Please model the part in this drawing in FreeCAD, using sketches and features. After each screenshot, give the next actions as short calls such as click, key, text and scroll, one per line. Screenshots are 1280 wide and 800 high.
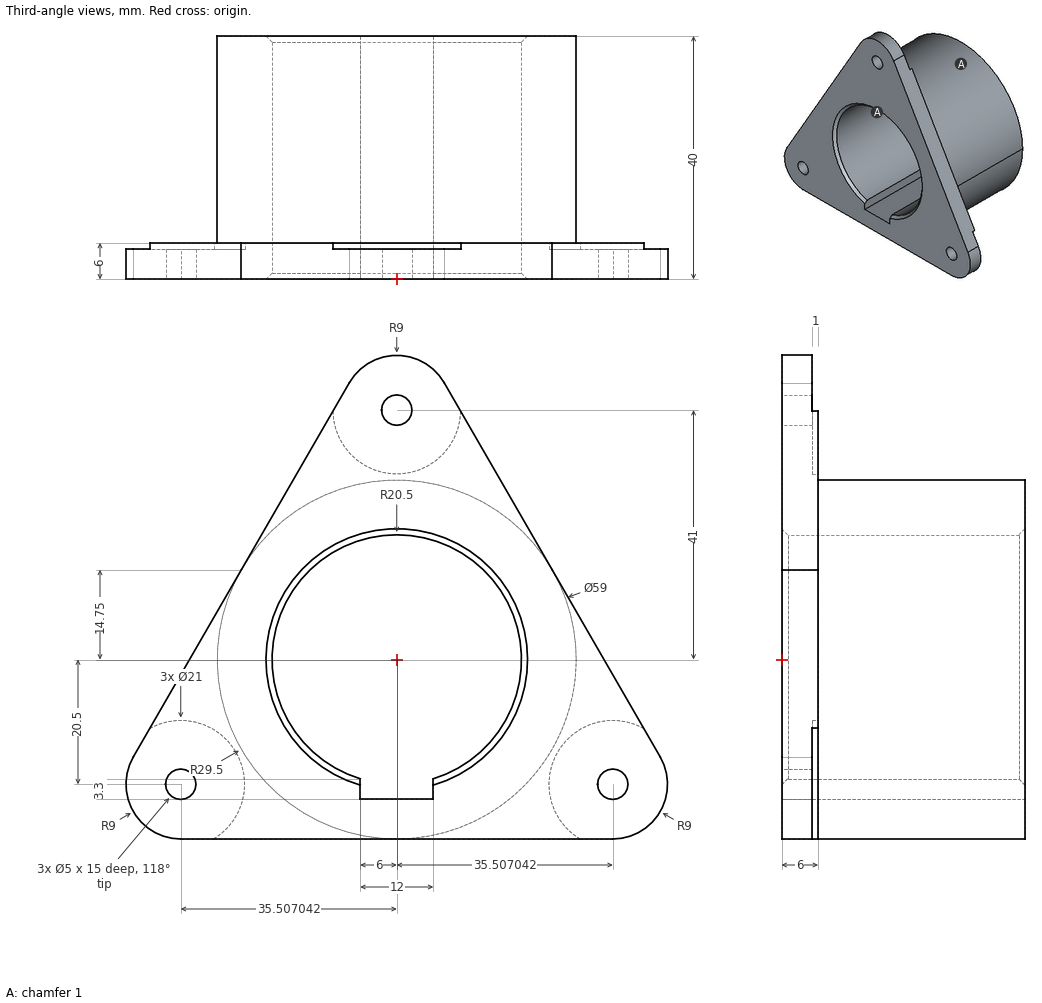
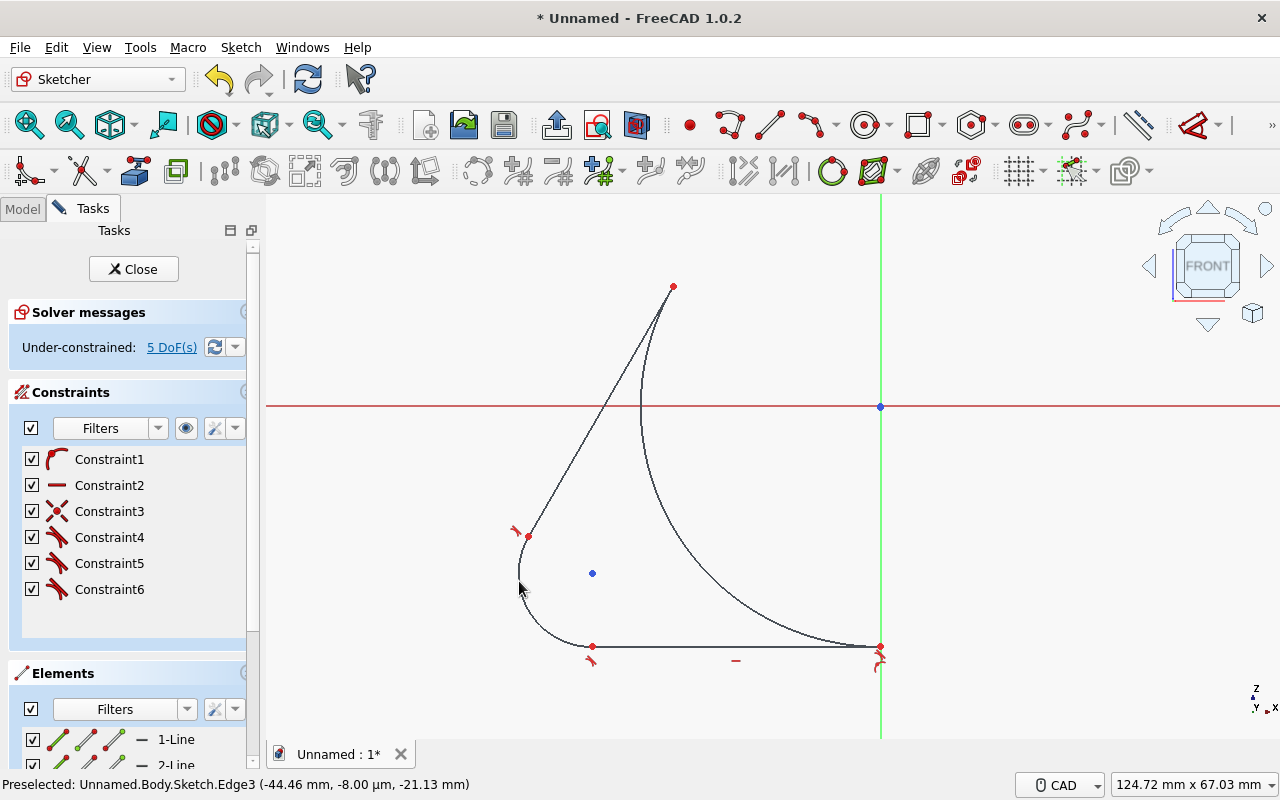
click(572, 462)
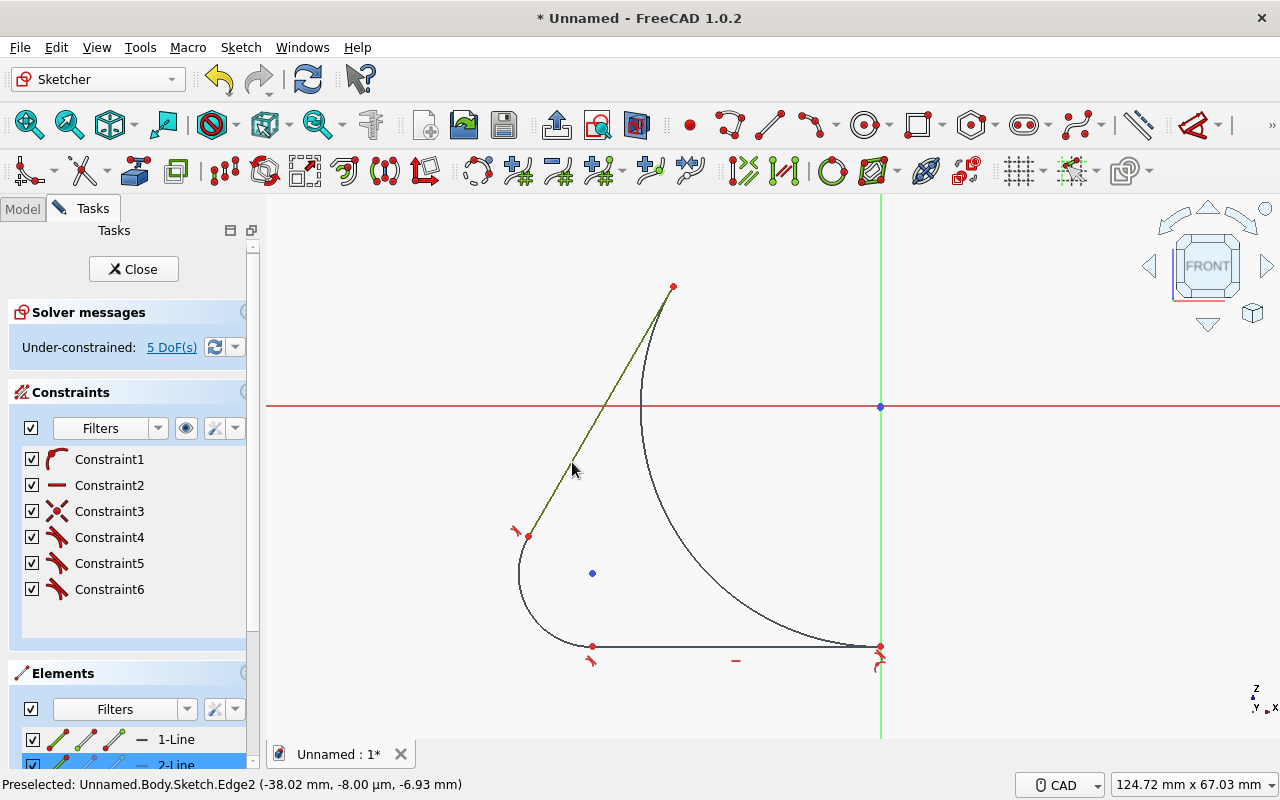
click(642, 432)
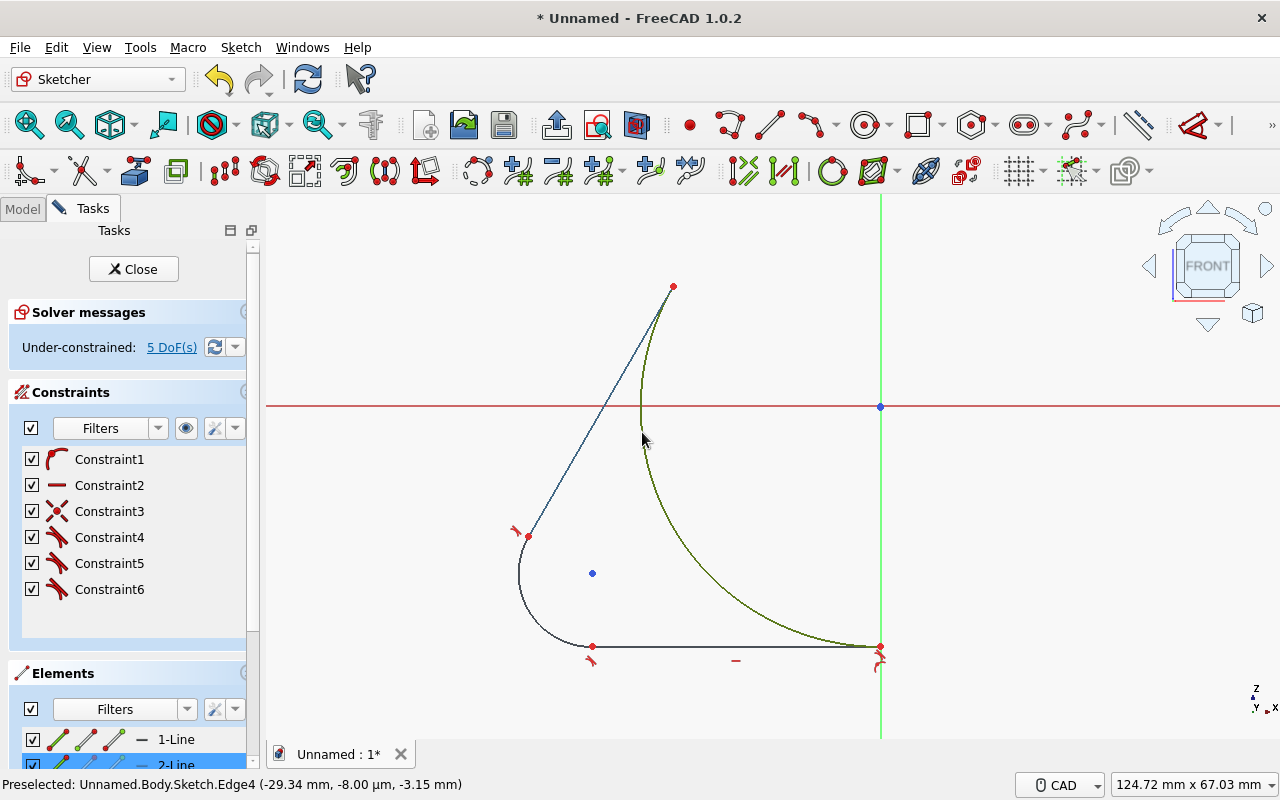
key(t)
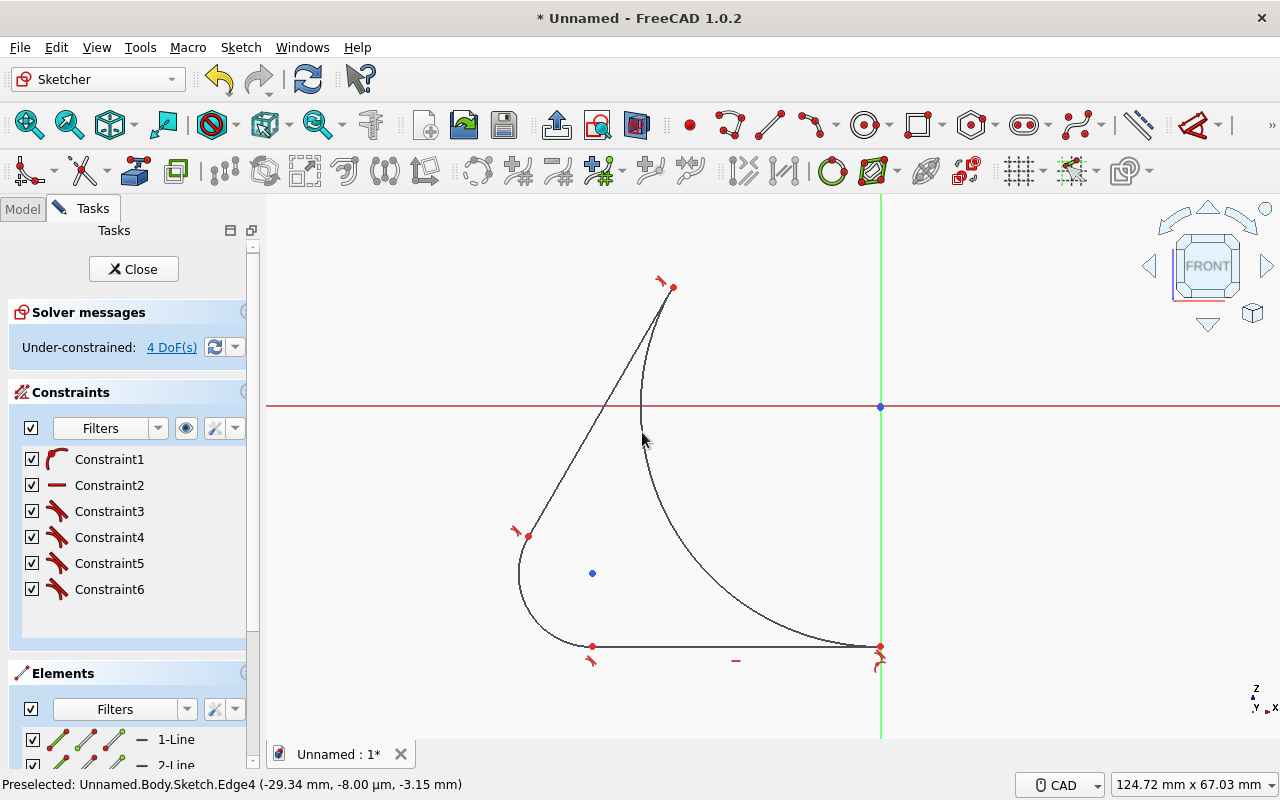
click(881, 407)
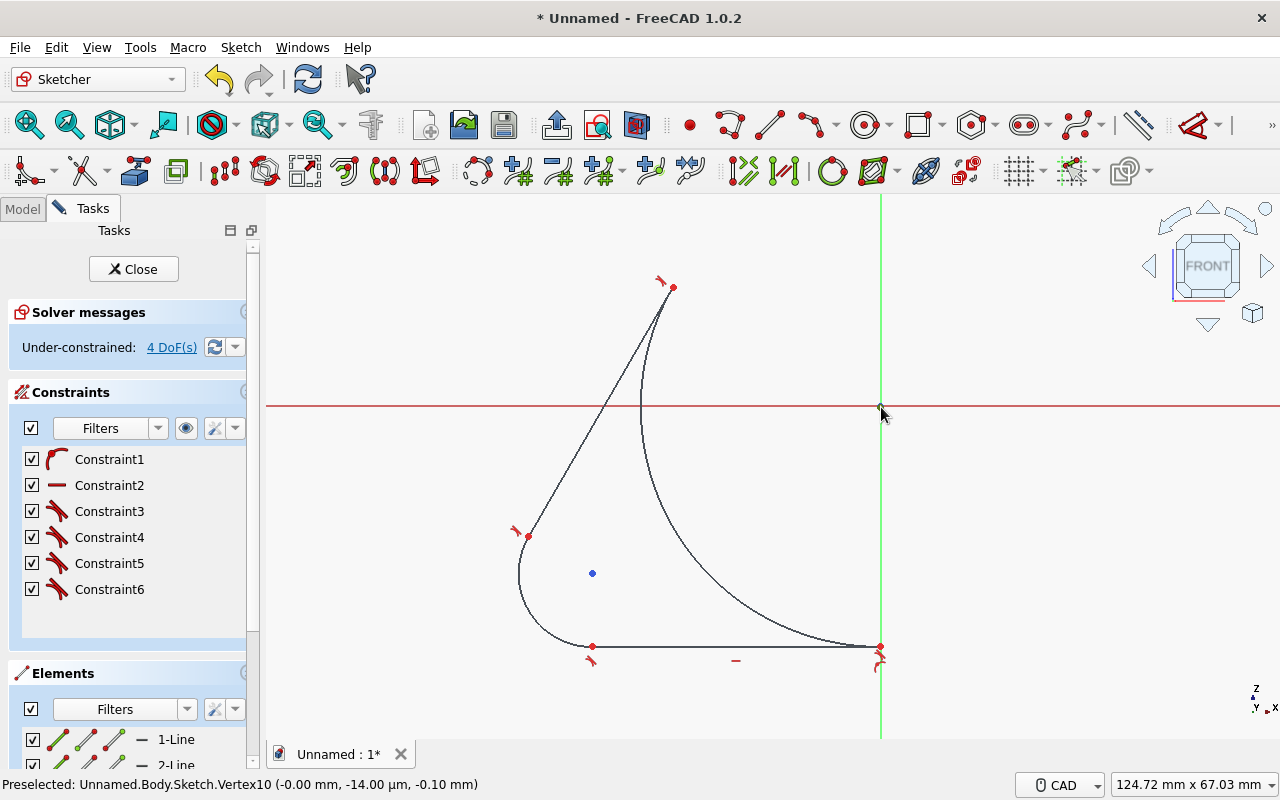
click(353, 406)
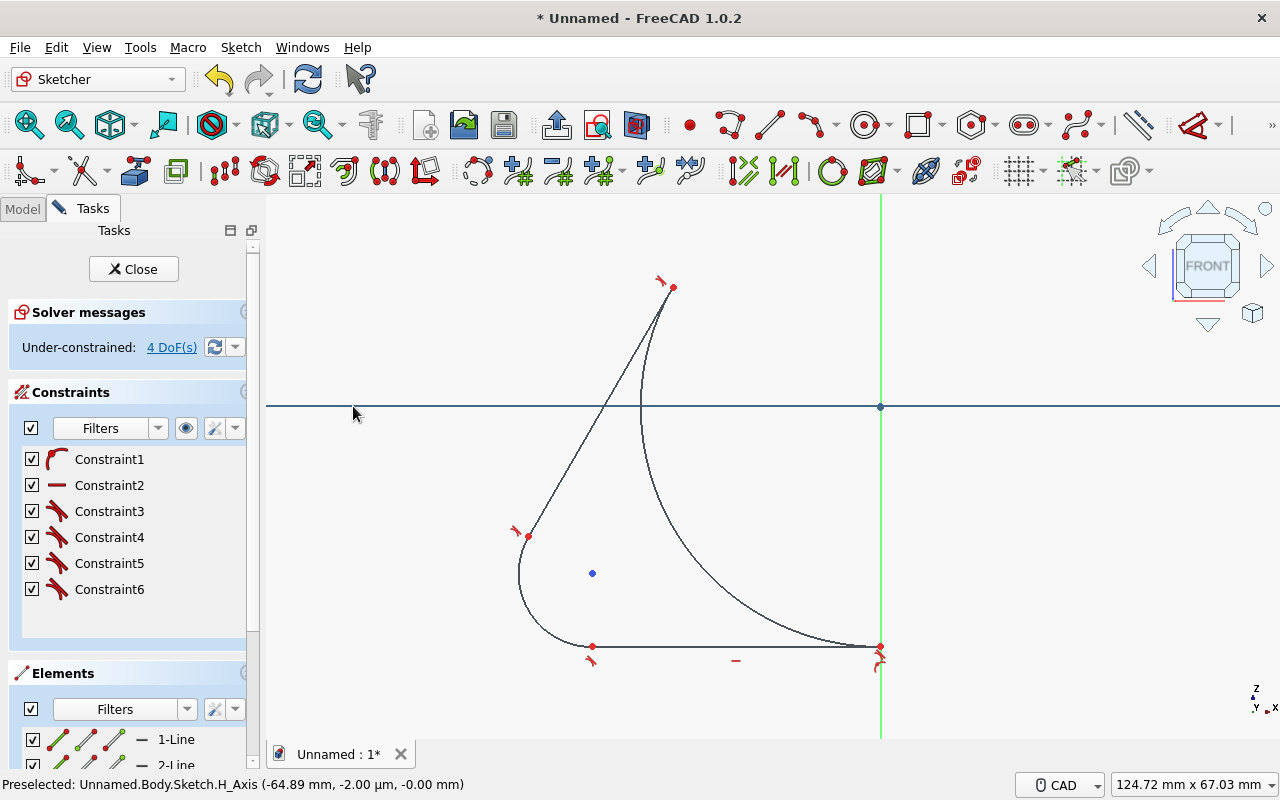
key(c)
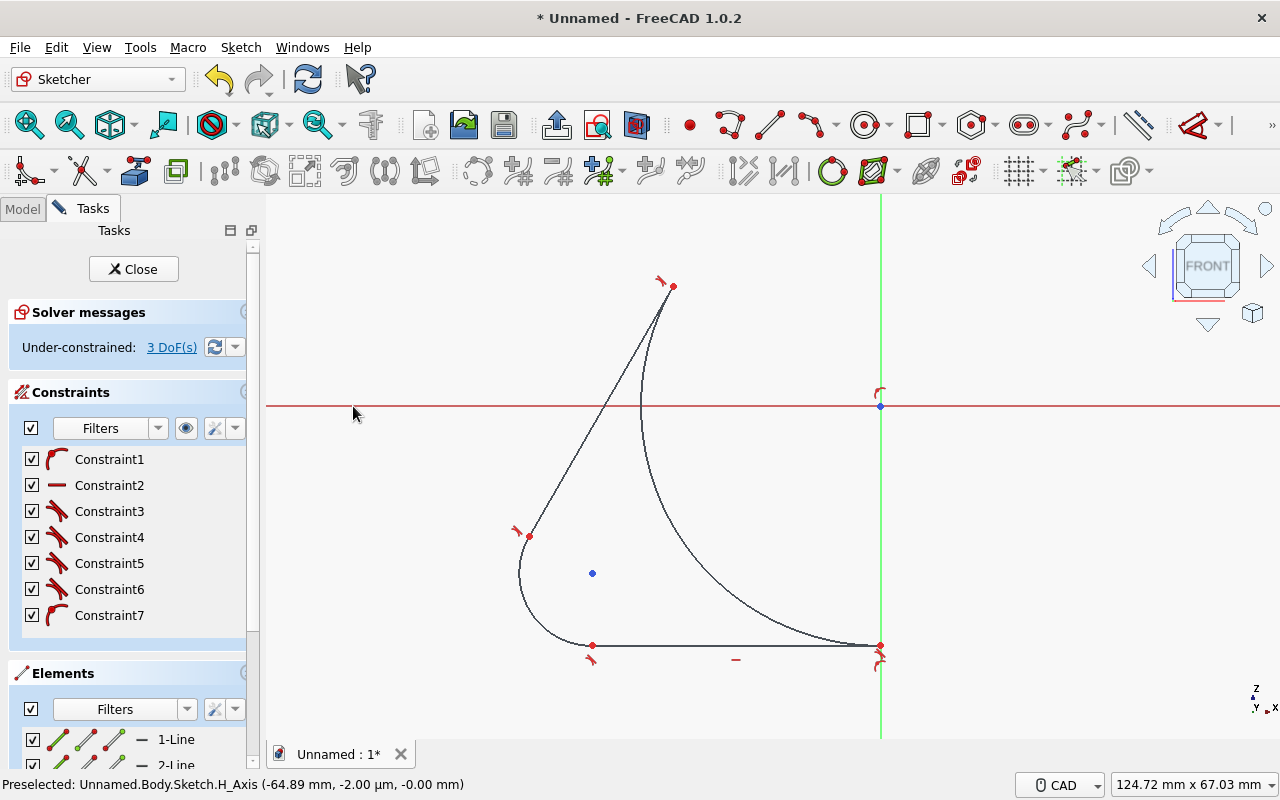
click(520, 581)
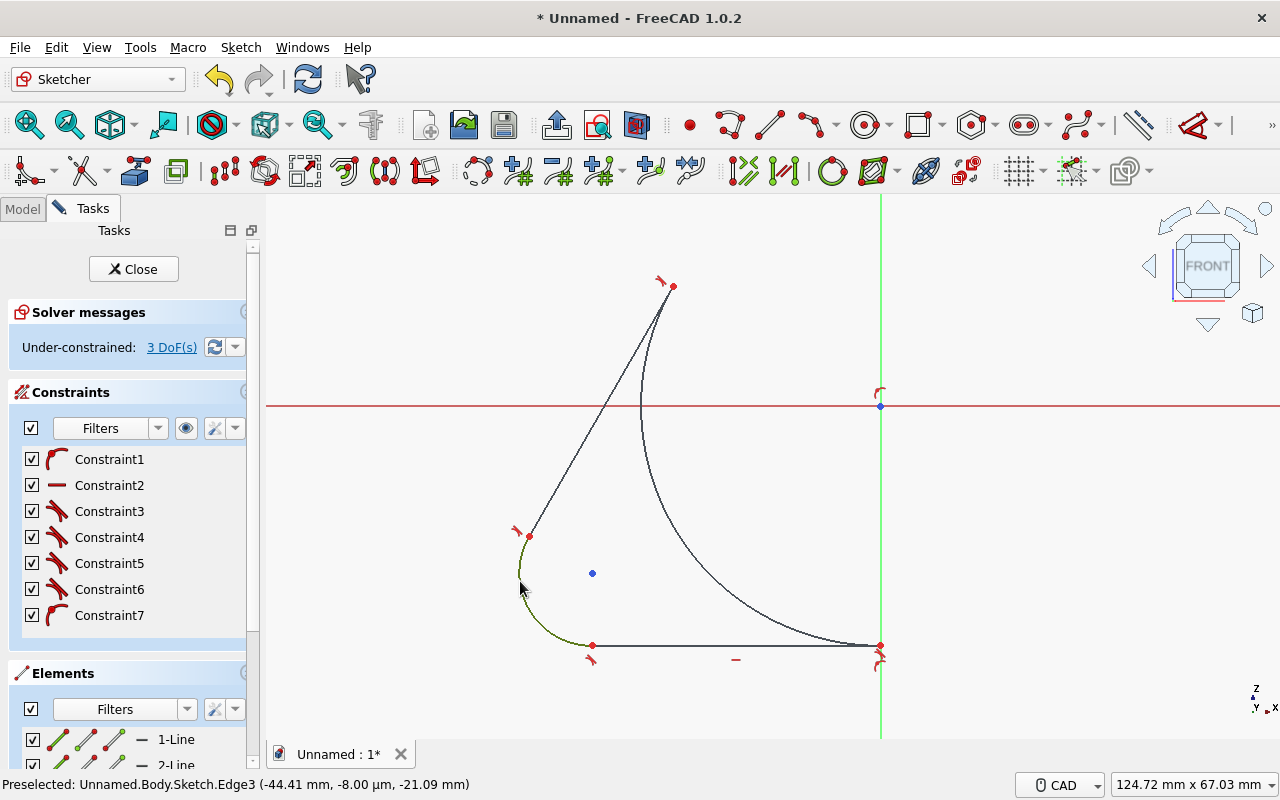
key(k)
key(r)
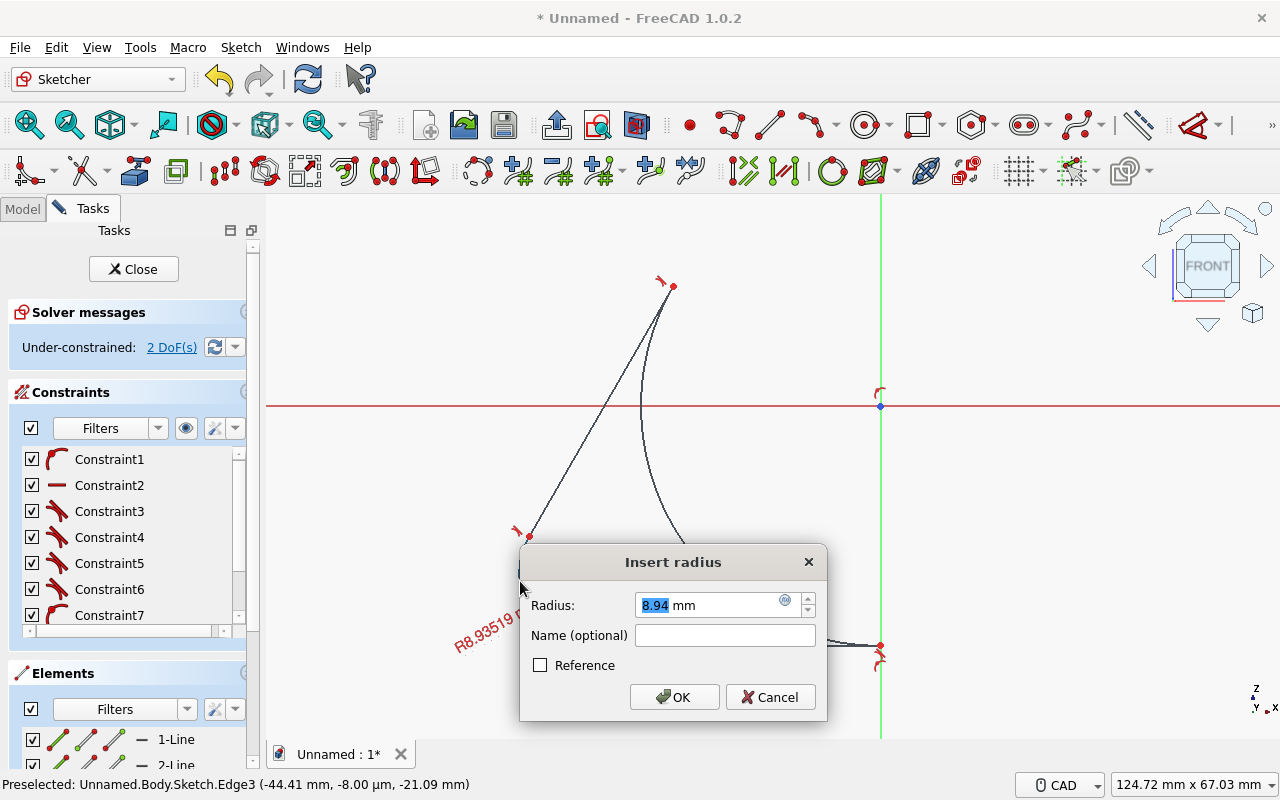
text(9)
key(Return)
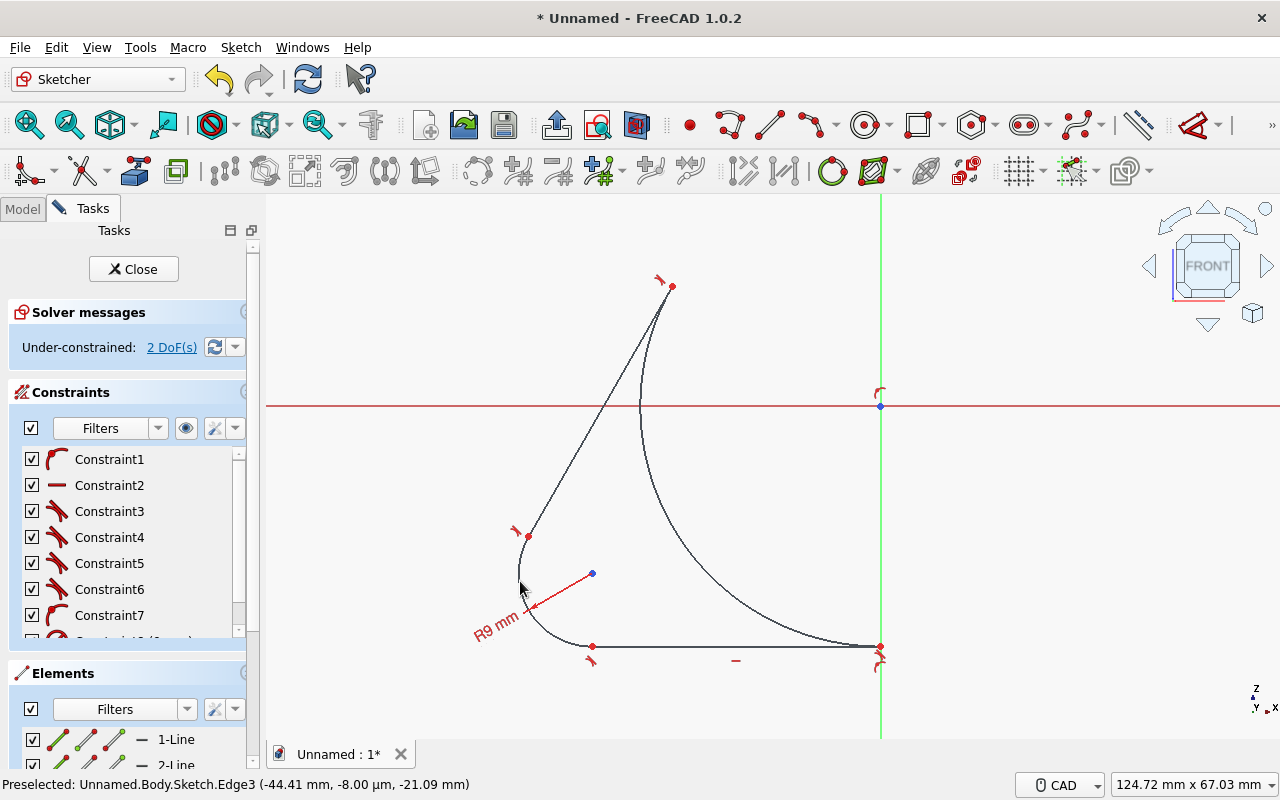
click(642, 432)